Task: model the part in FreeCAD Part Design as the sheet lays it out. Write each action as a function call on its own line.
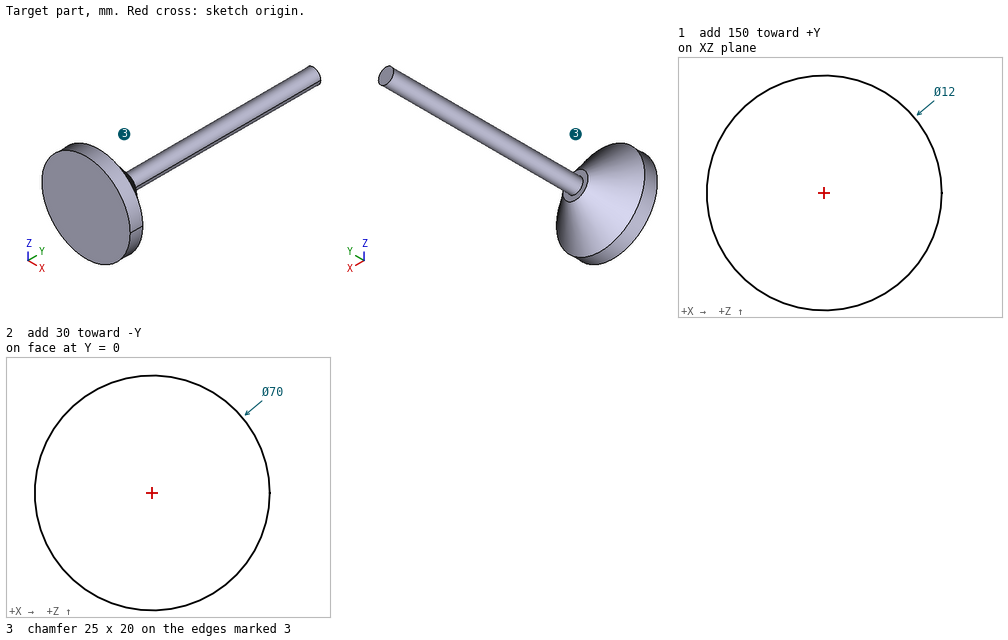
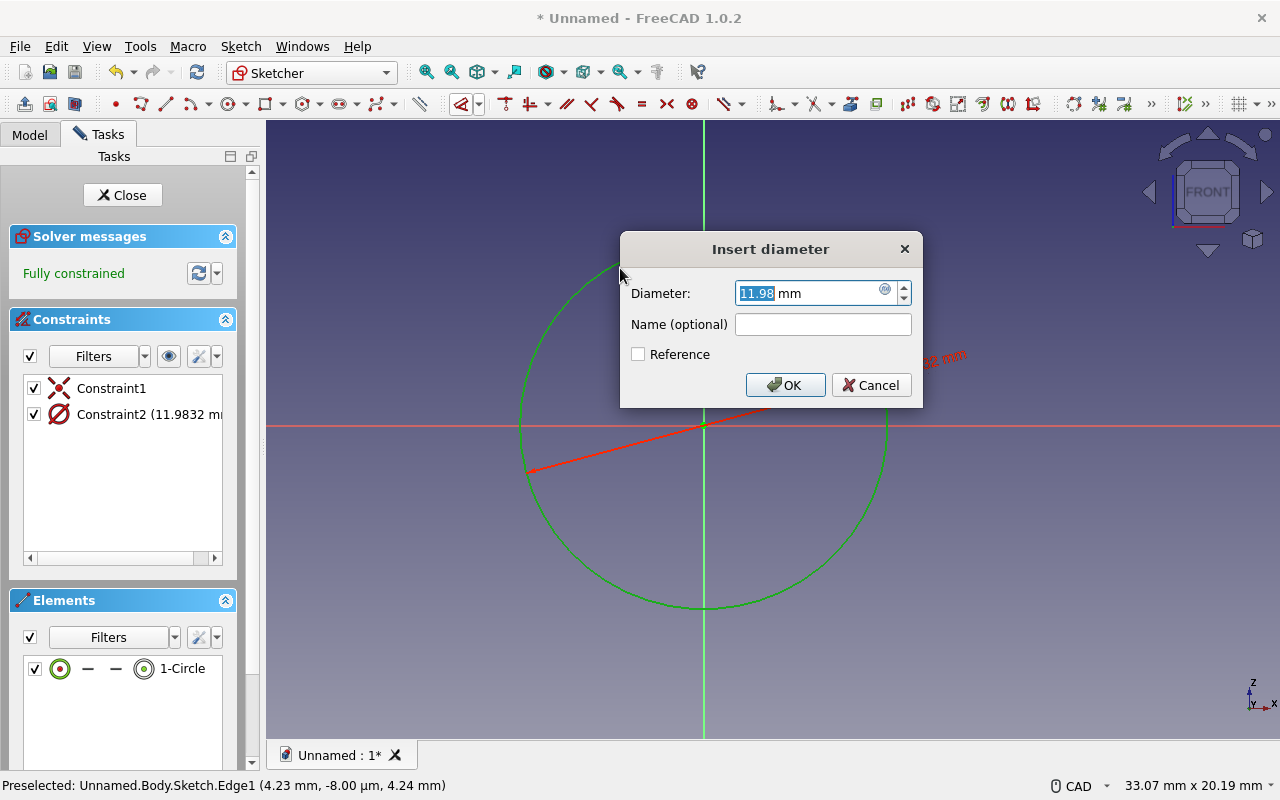
text(12)
key(Return)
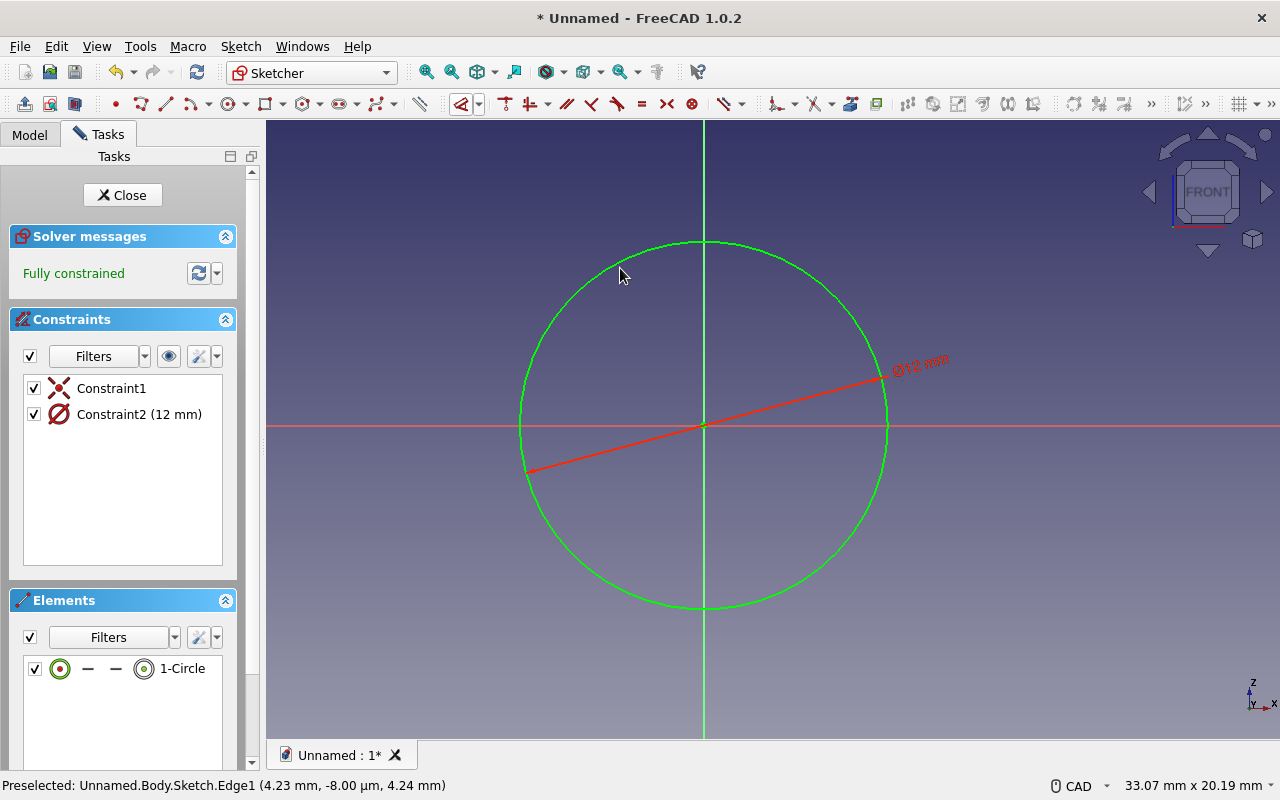
click(123, 195)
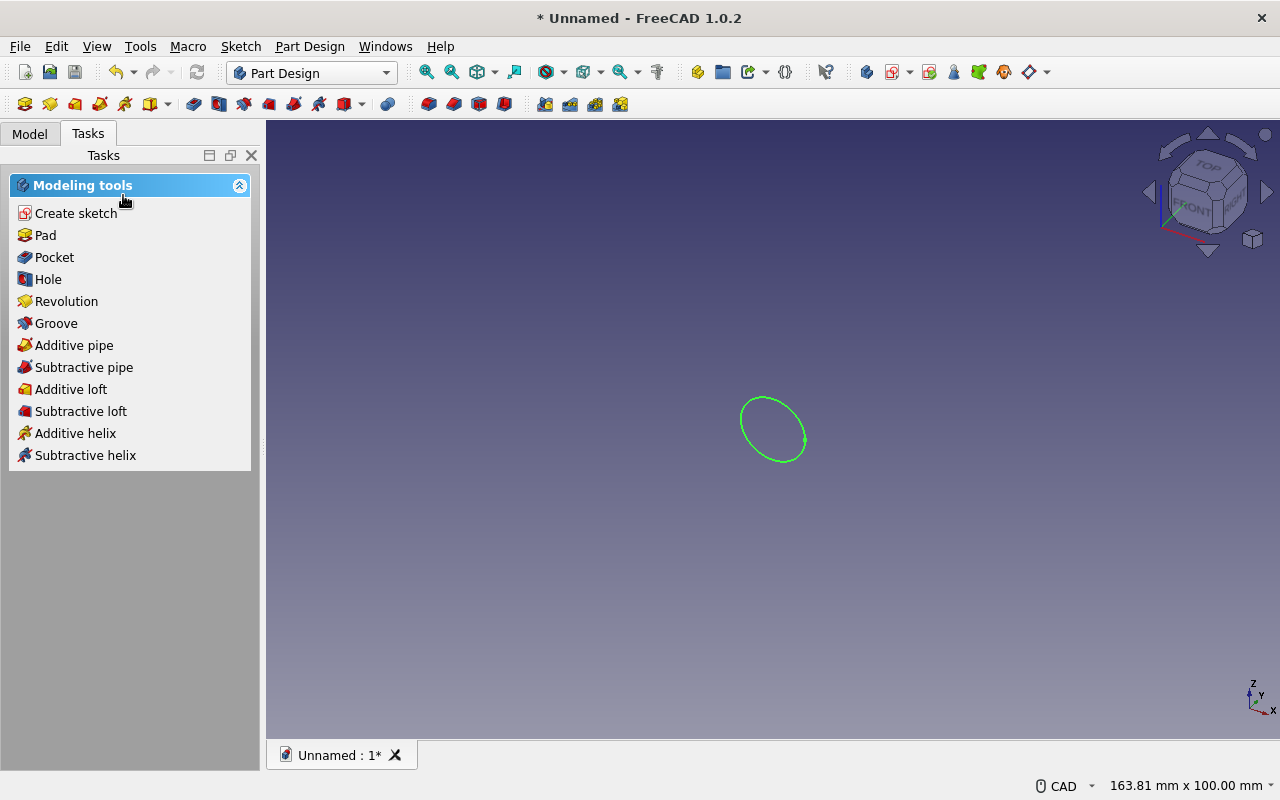
click(25, 104)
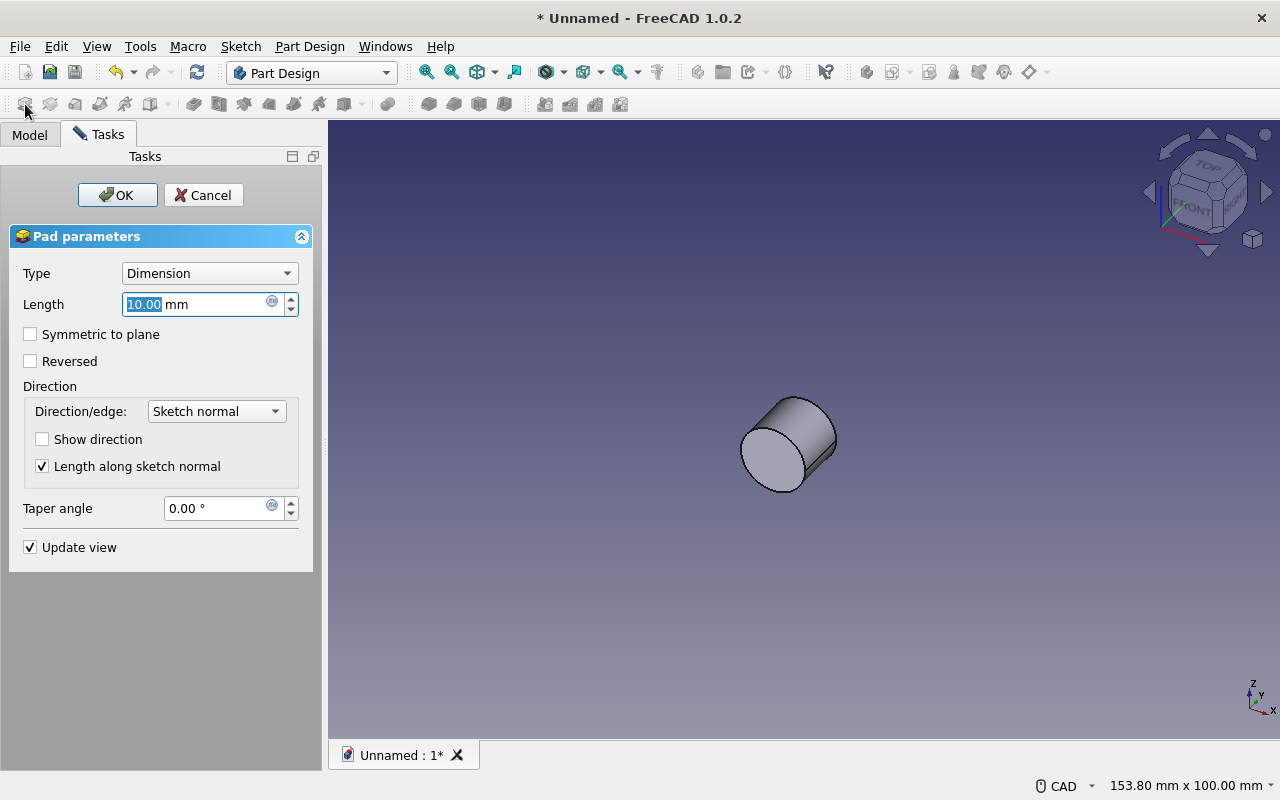
text(150)
key(Tab)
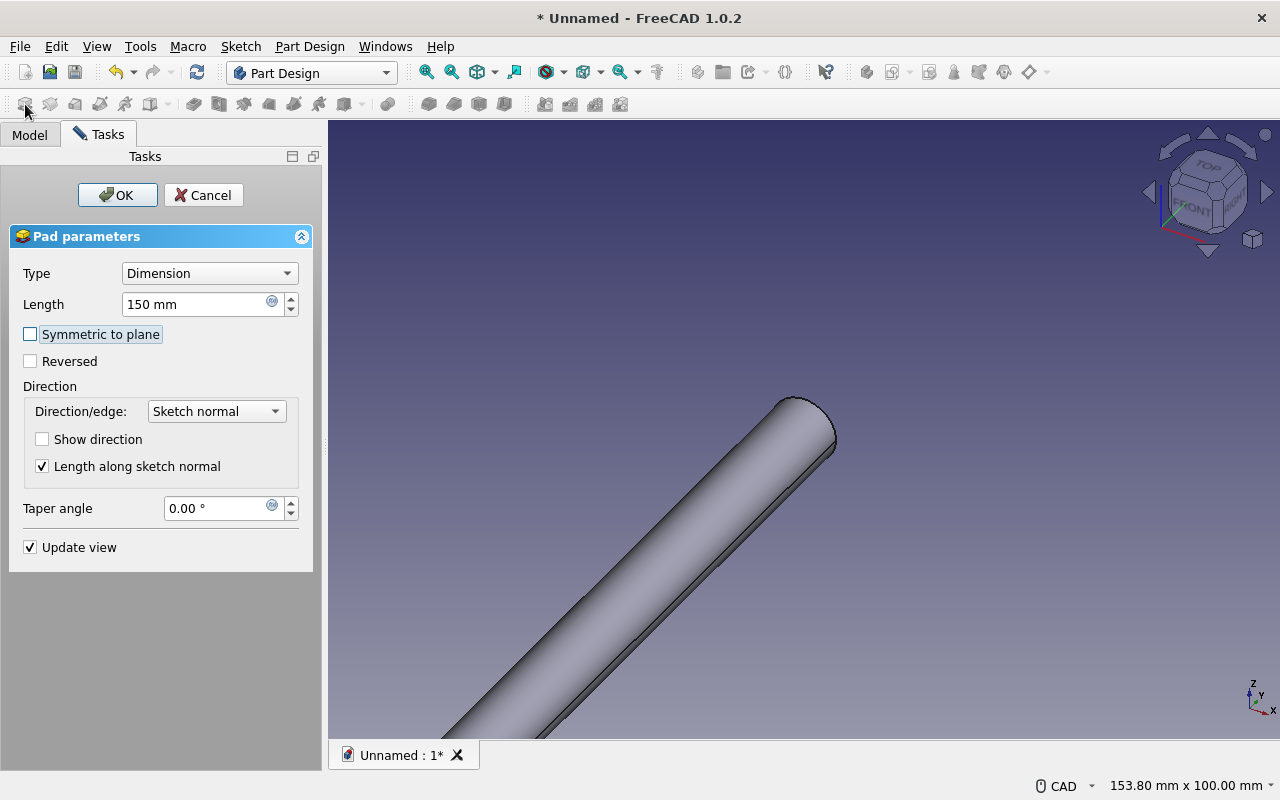
click(31, 361)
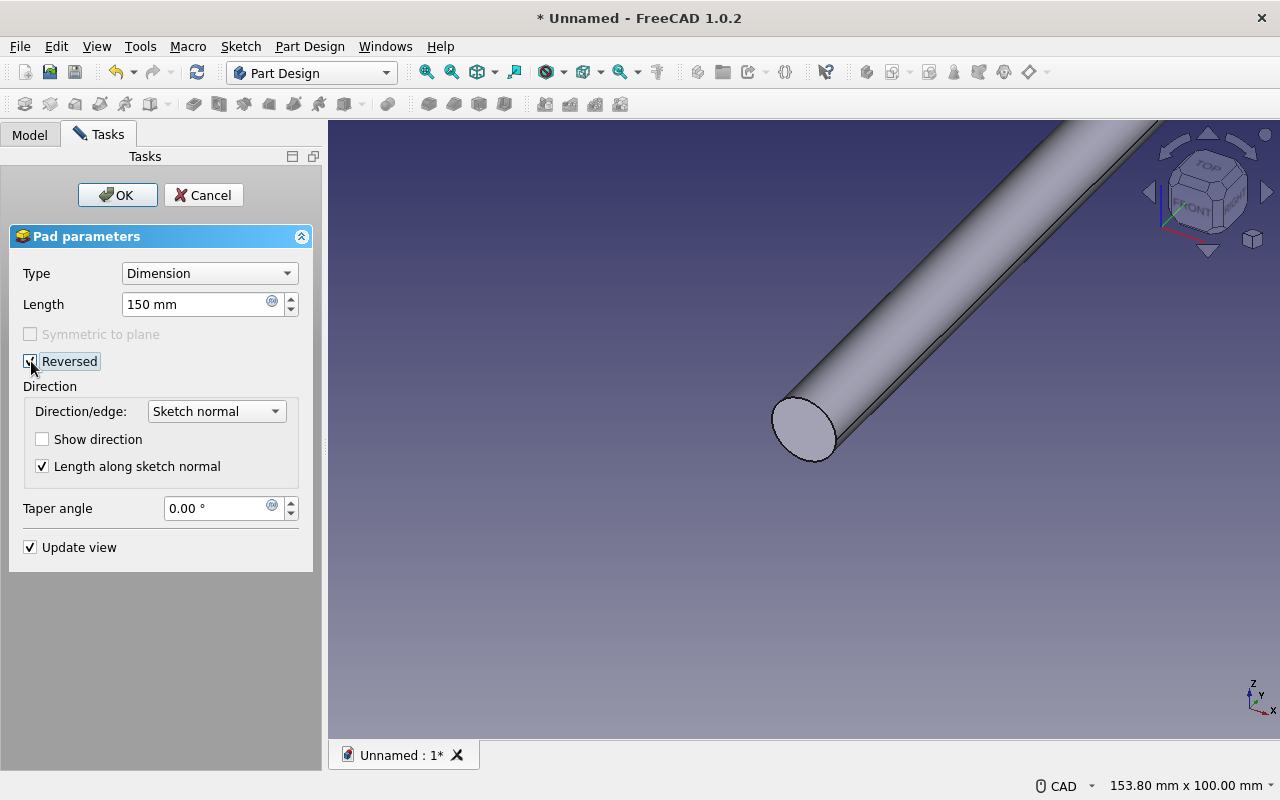
click(118, 195)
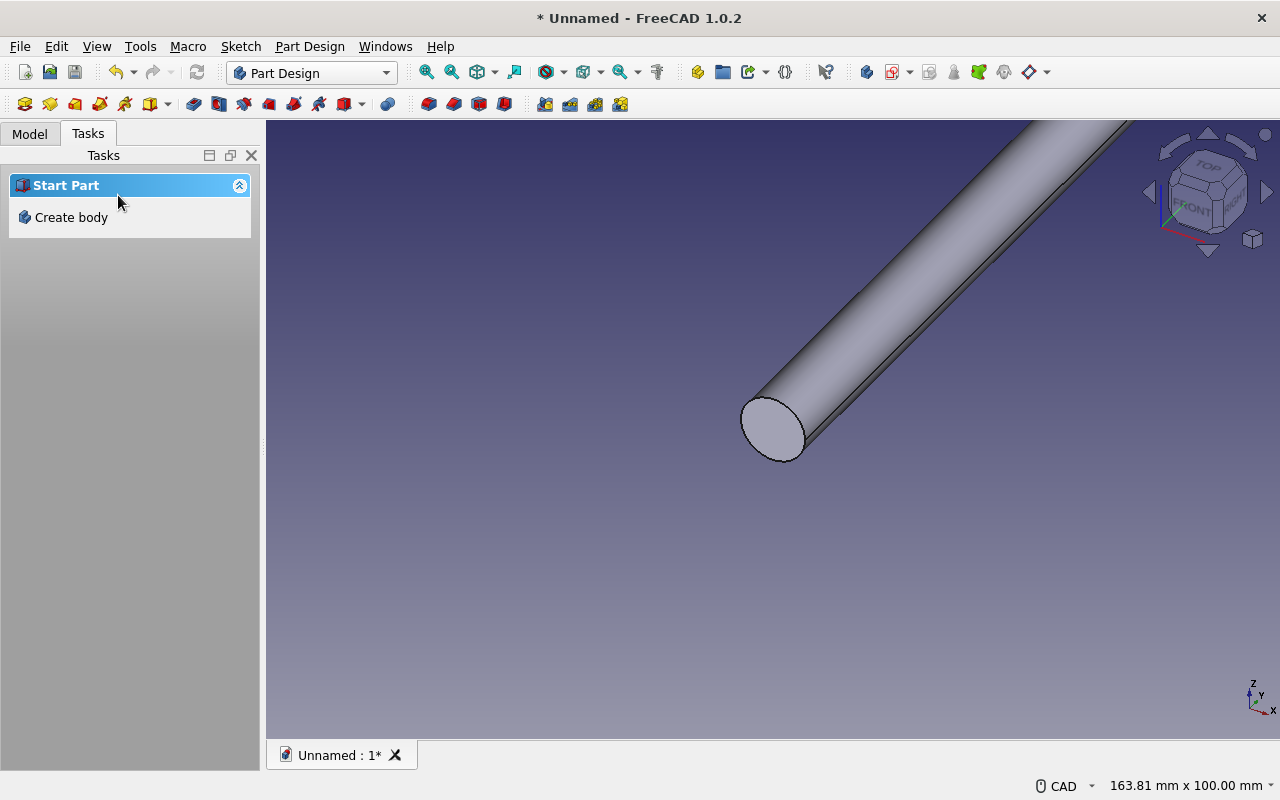
click(427, 72)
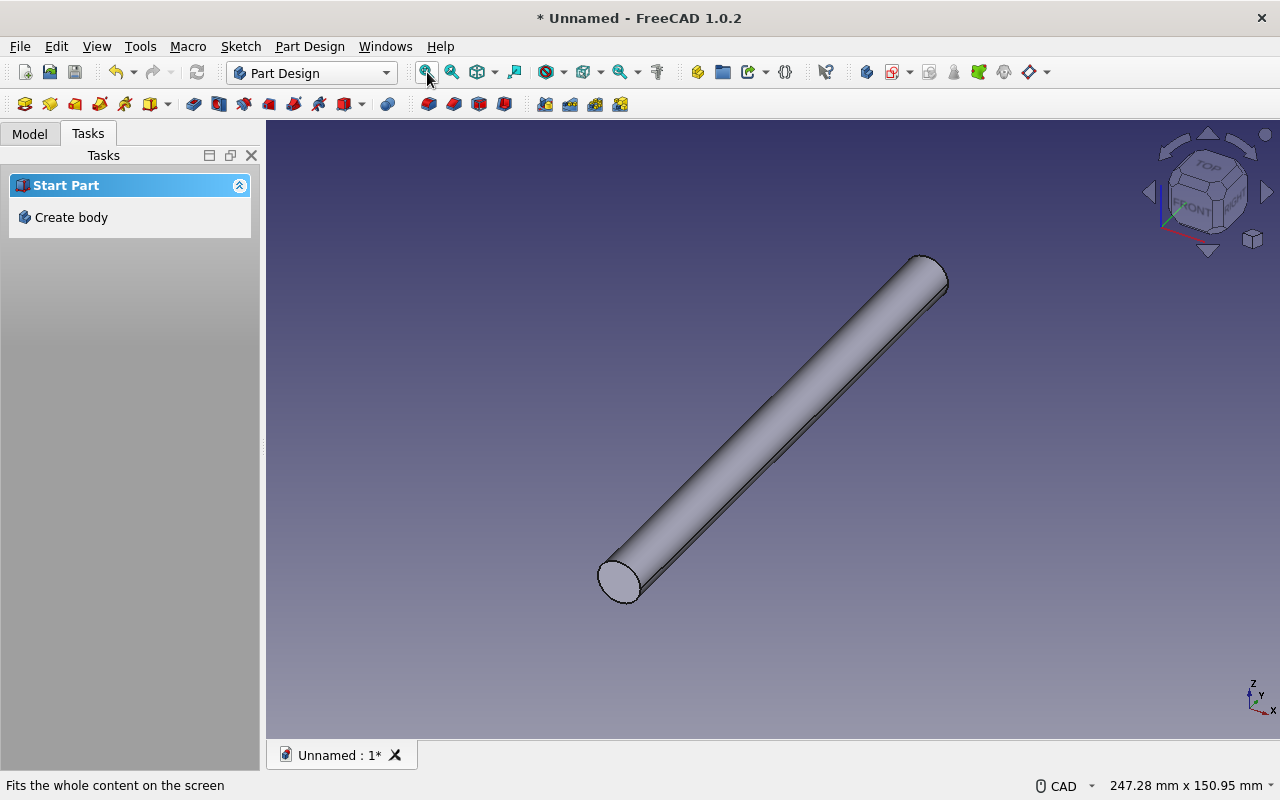
click(619, 581)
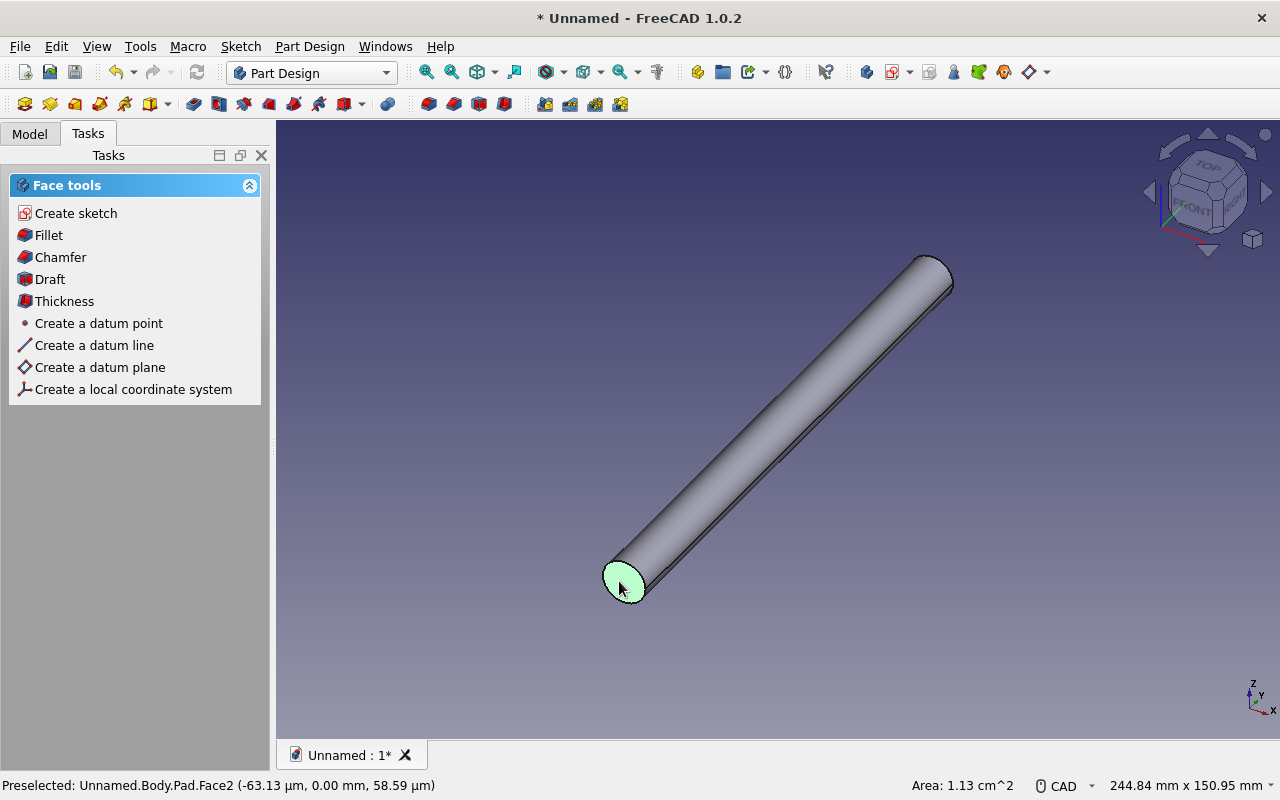
click(892, 72)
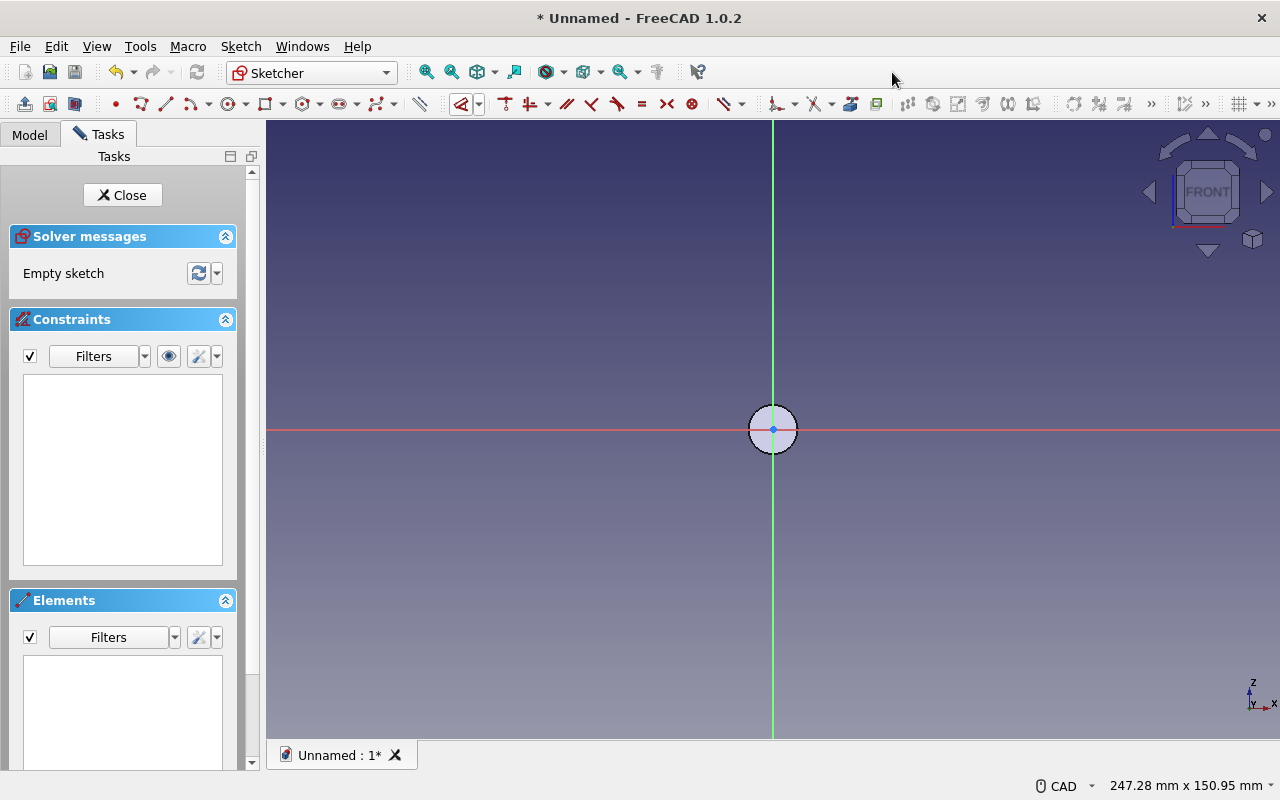
scroll(912, 430, up, 2)